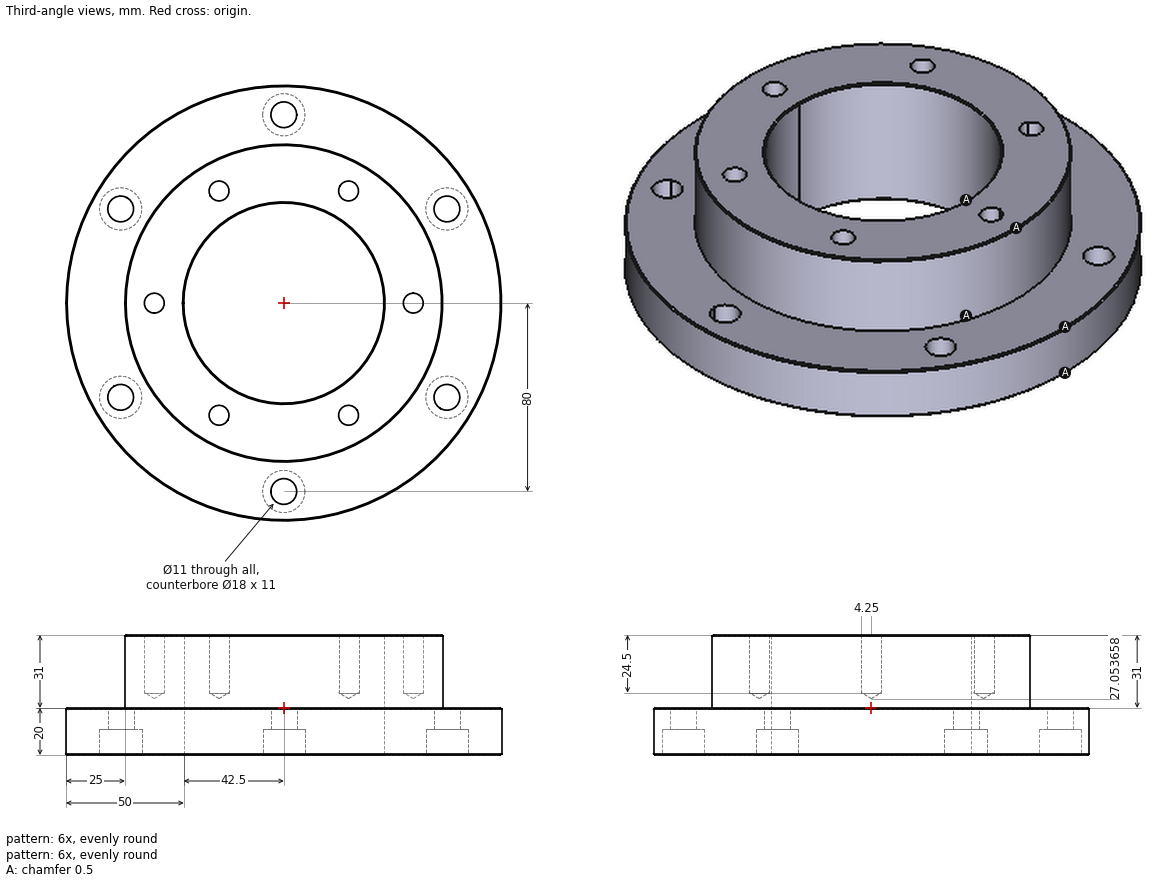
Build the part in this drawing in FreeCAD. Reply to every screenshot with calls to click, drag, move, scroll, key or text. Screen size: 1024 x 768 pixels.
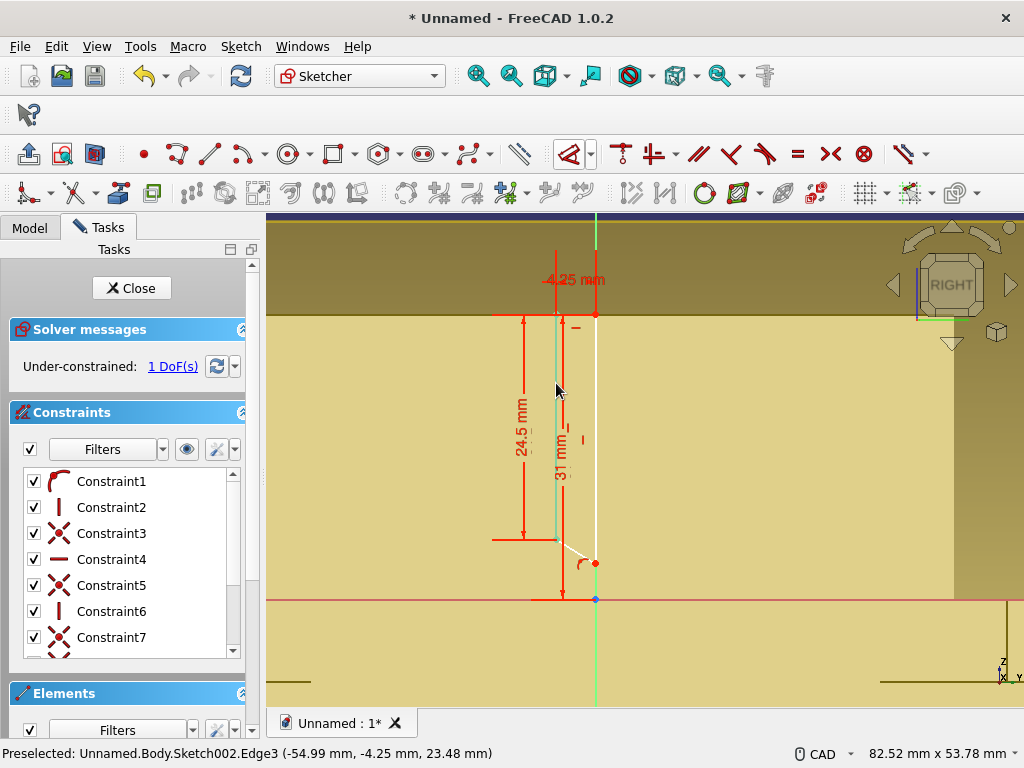
click(596, 489)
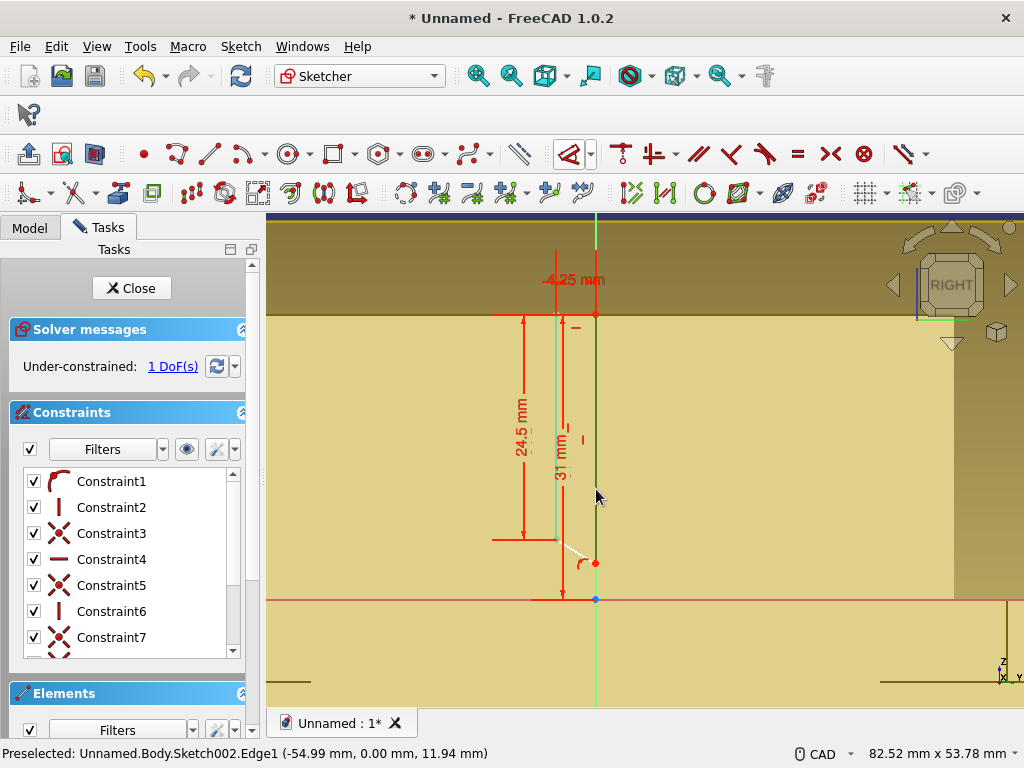
key(i)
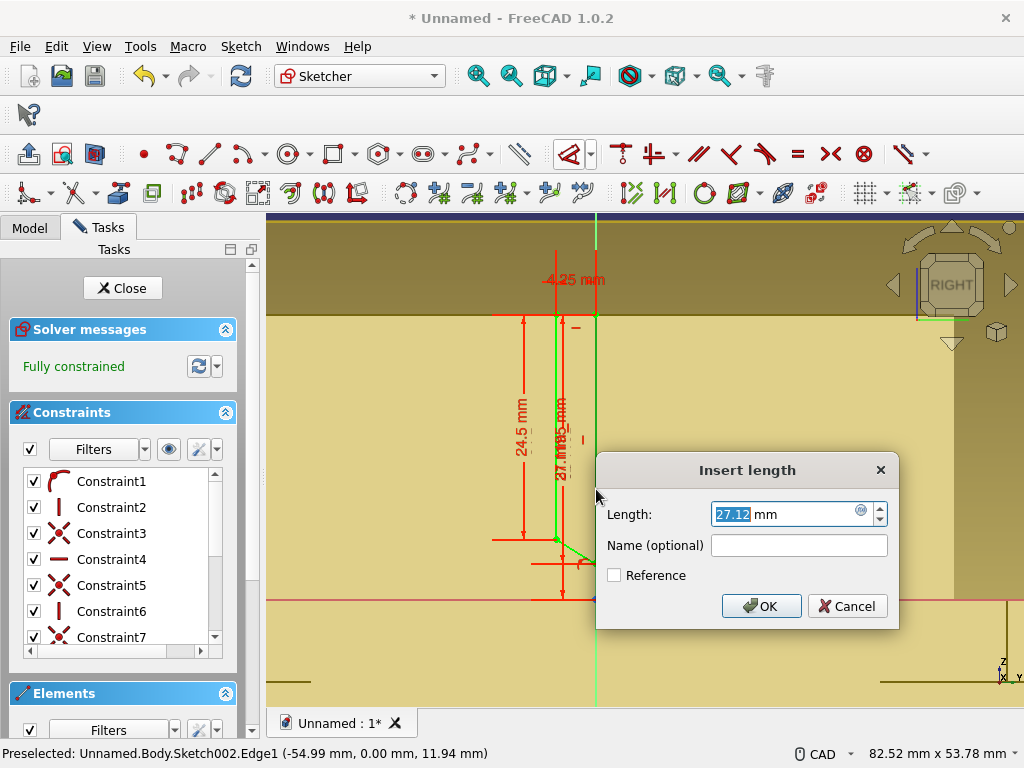
text(27.053658)
key(Return)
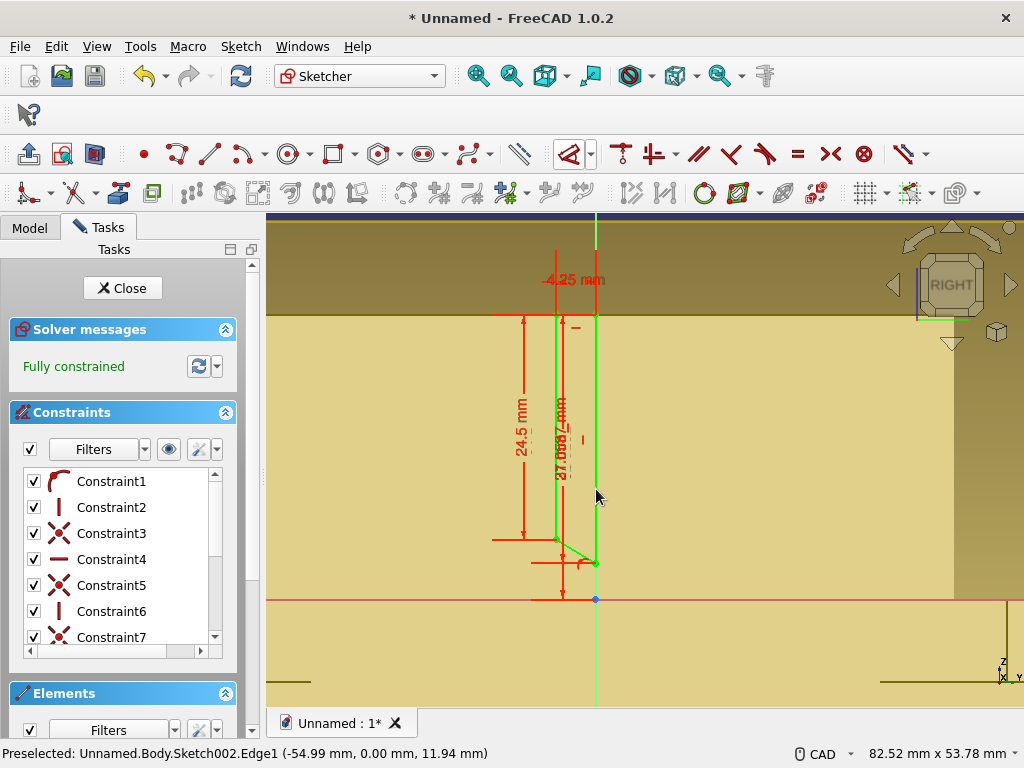
click(123, 288)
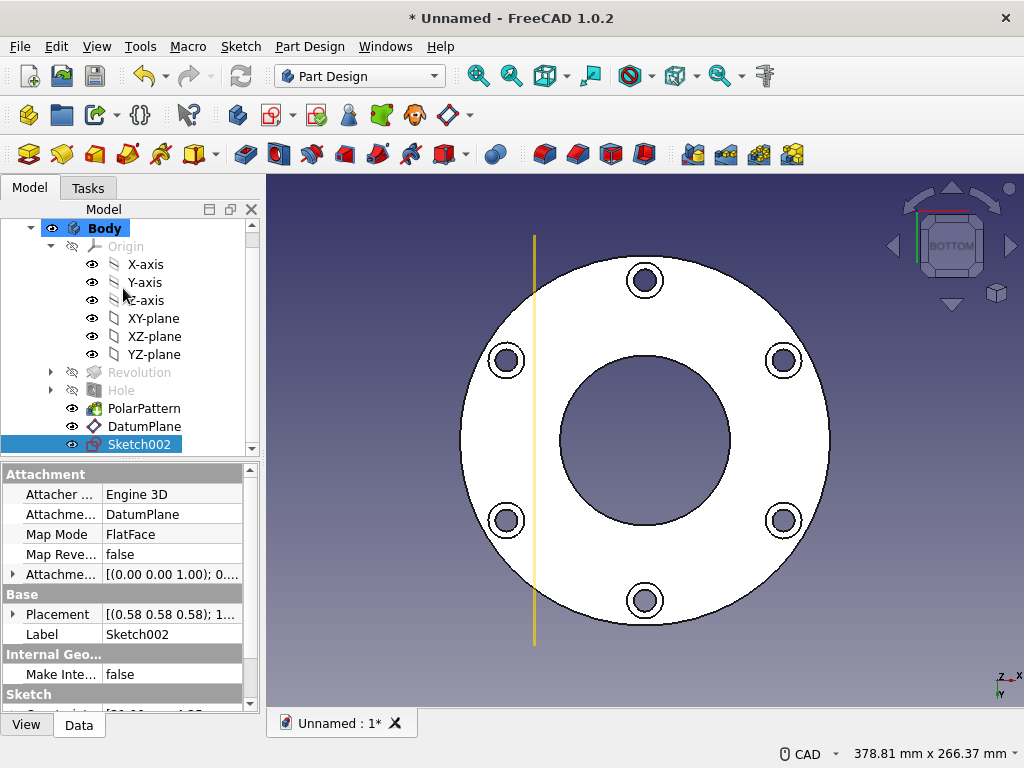
click(312, 154)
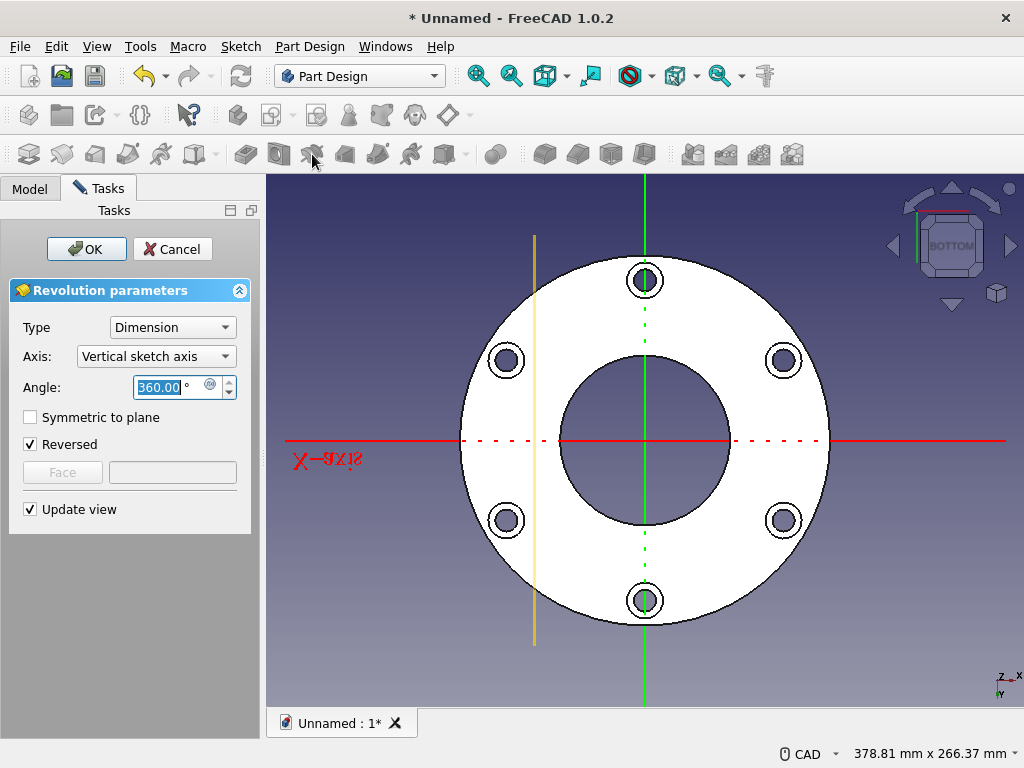
click(87, 249)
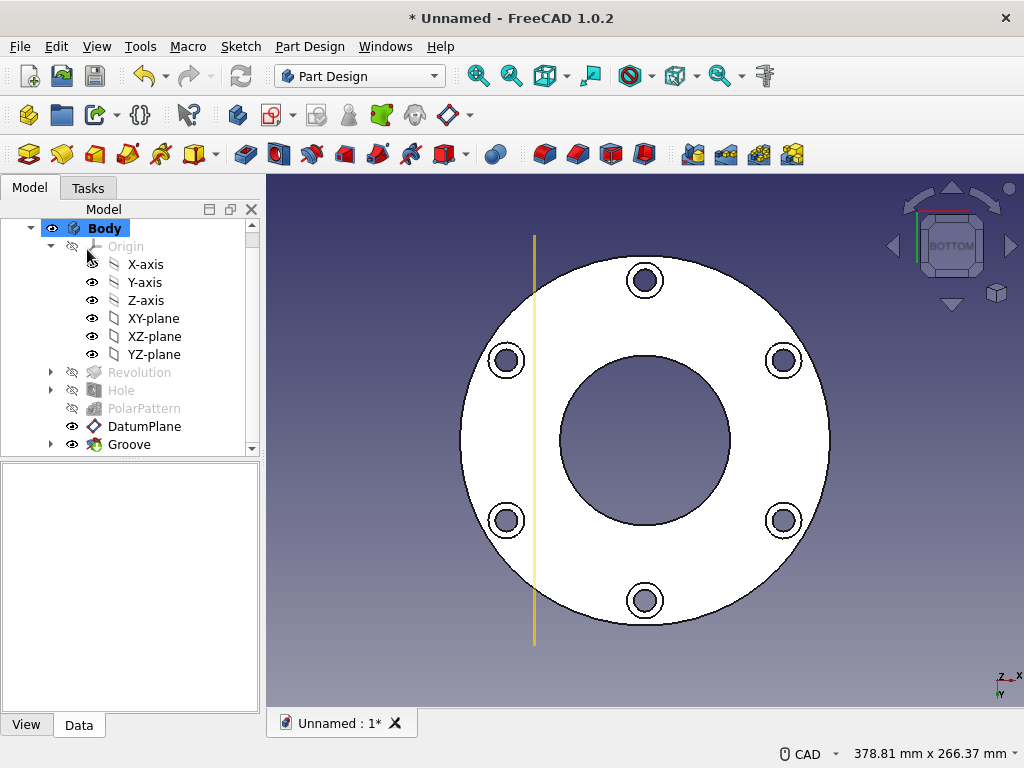
click(117, 426)
key(space)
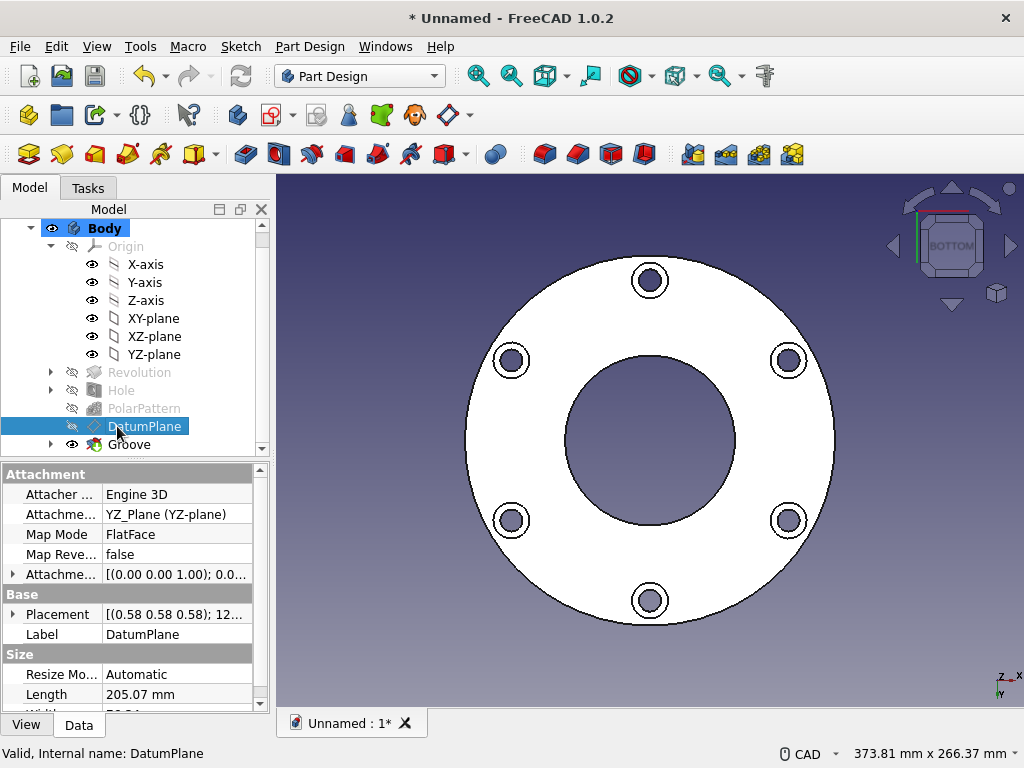
click(117, 444)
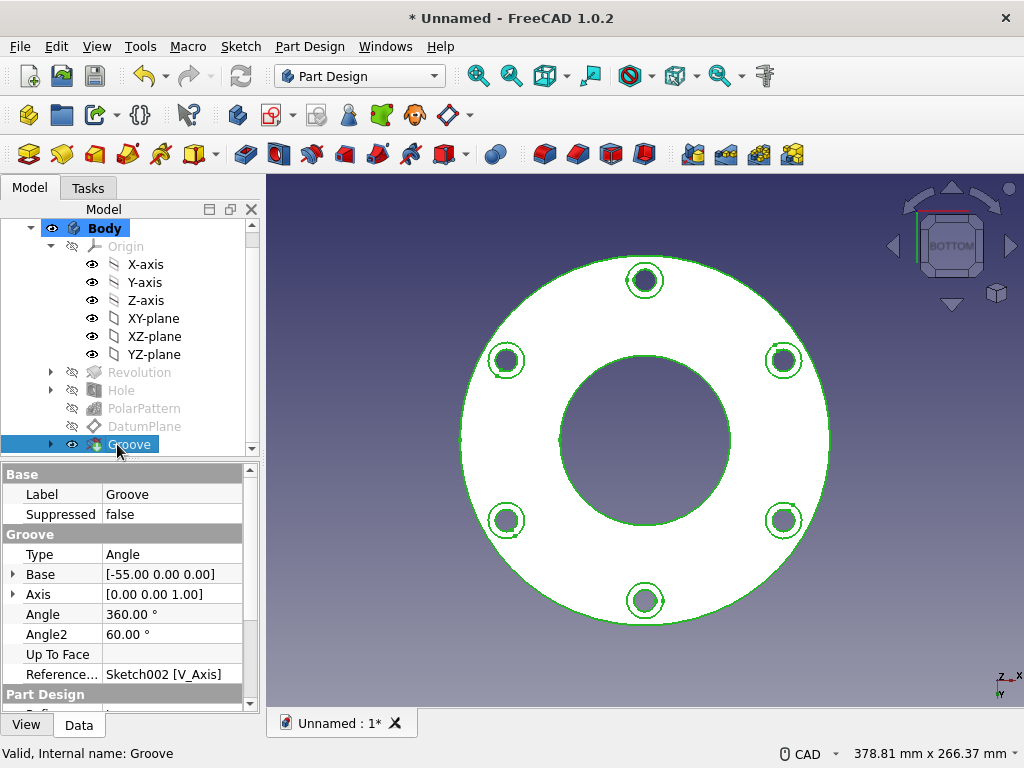
click(759, 154)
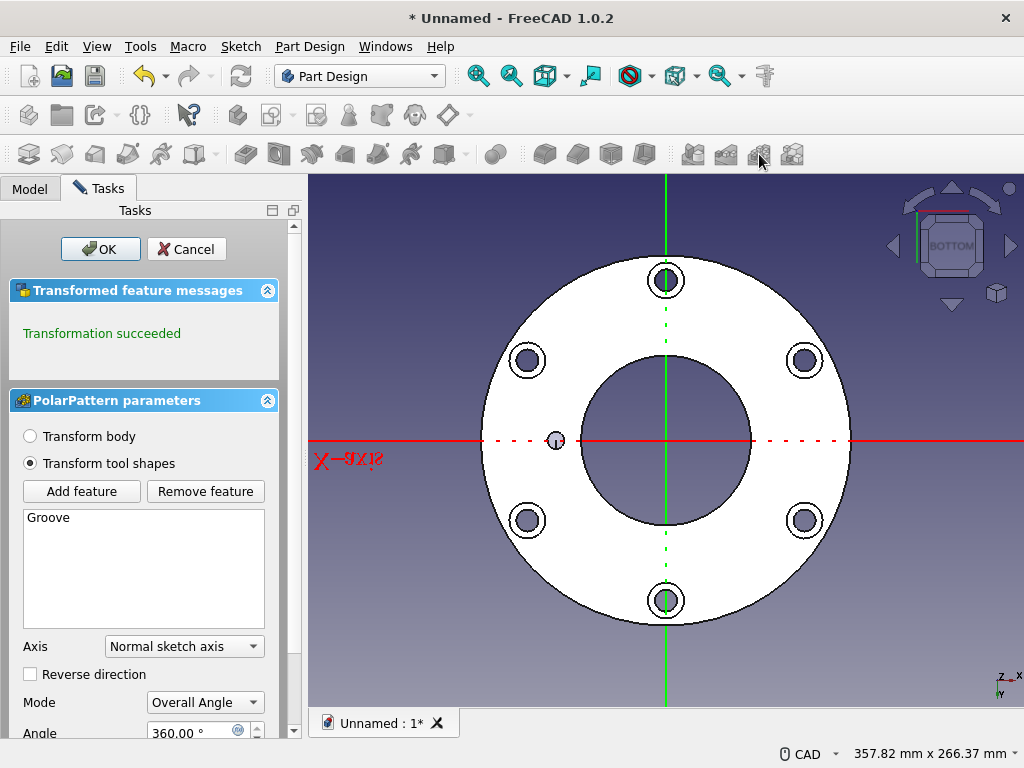
click(185, 646)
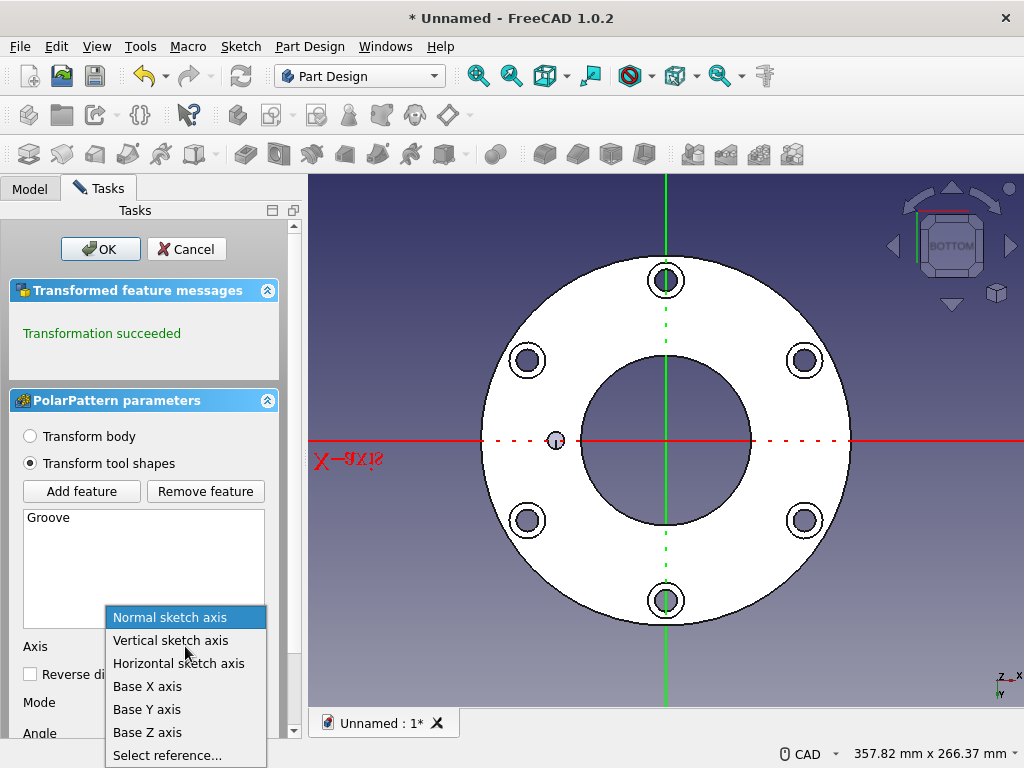
click(184, 732)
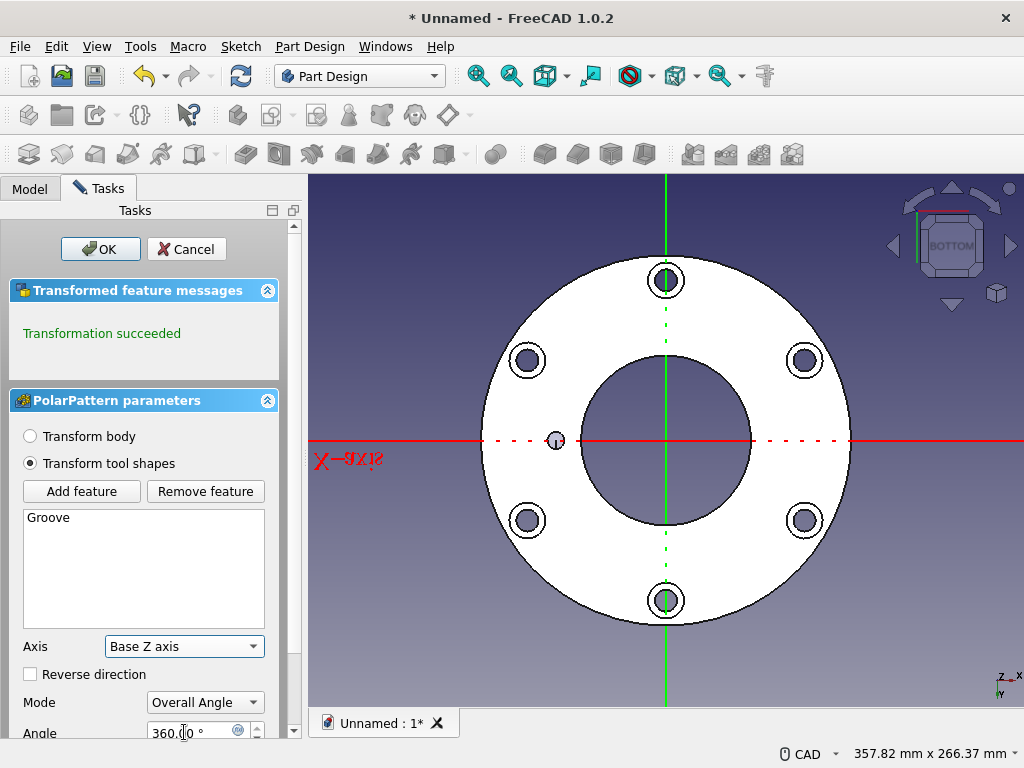
scroll(294, 479, down, 2)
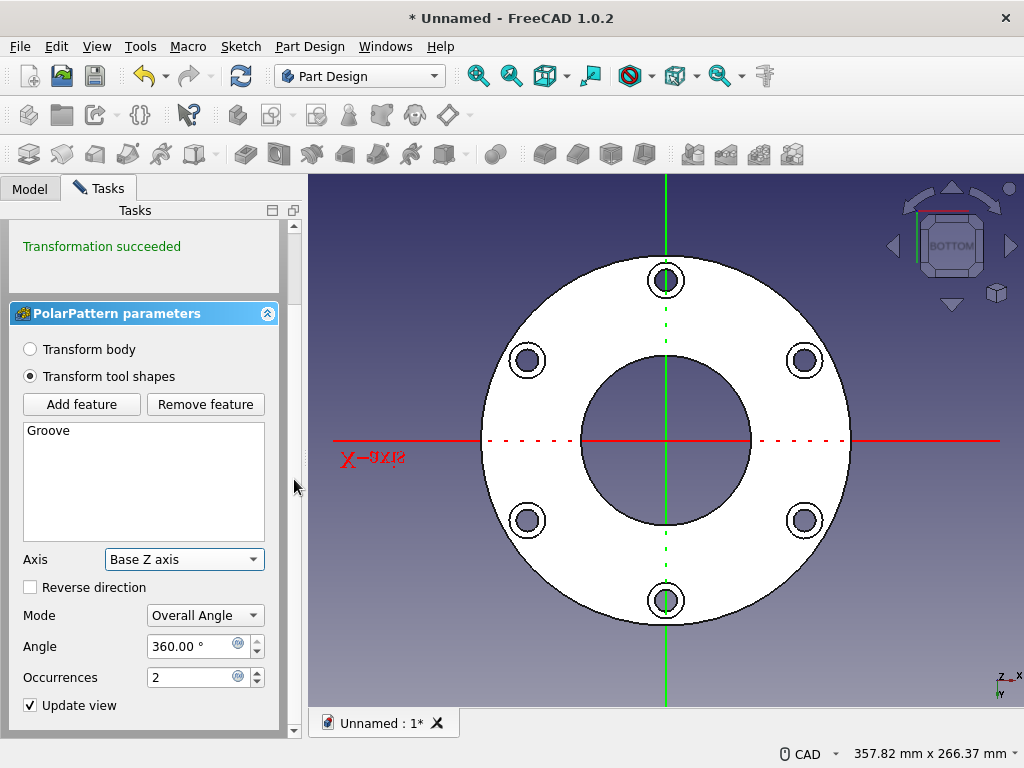
triple_click(199, 678)